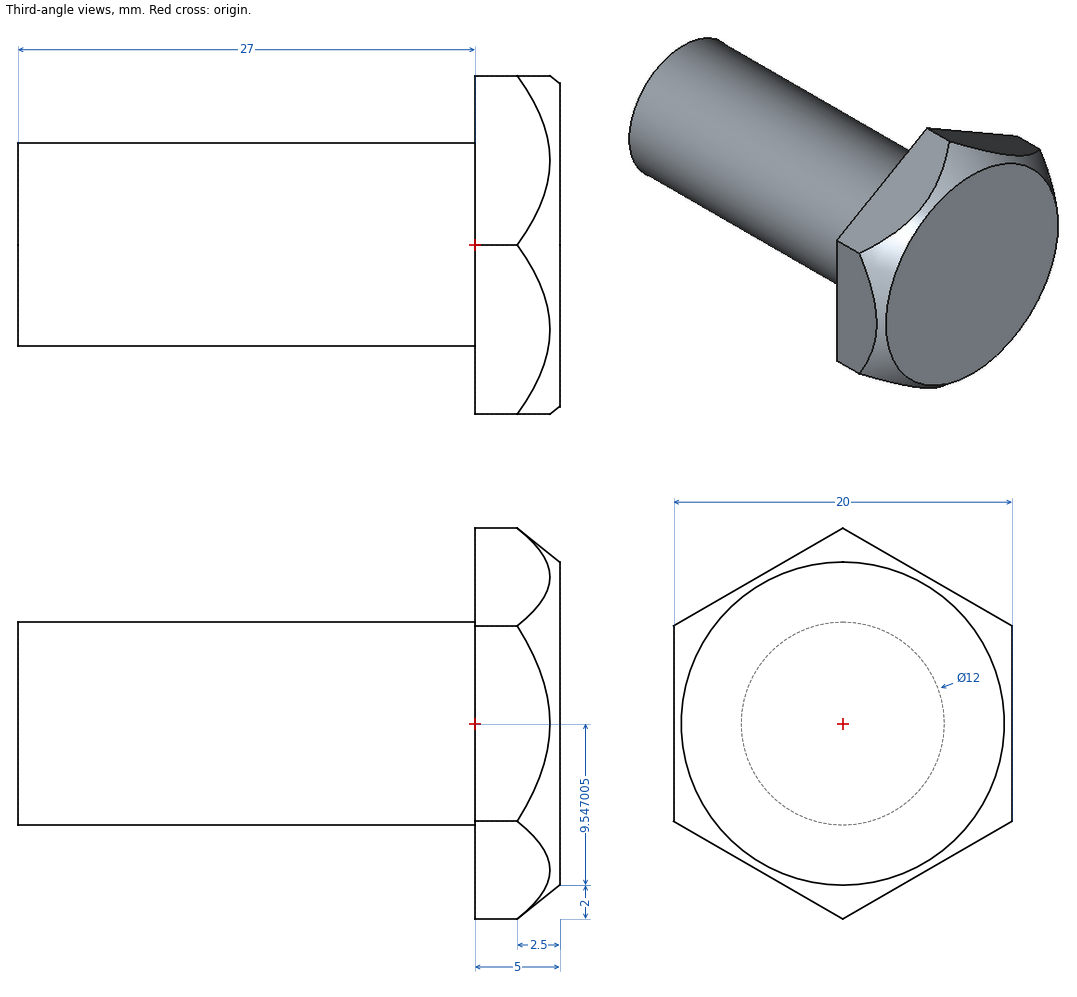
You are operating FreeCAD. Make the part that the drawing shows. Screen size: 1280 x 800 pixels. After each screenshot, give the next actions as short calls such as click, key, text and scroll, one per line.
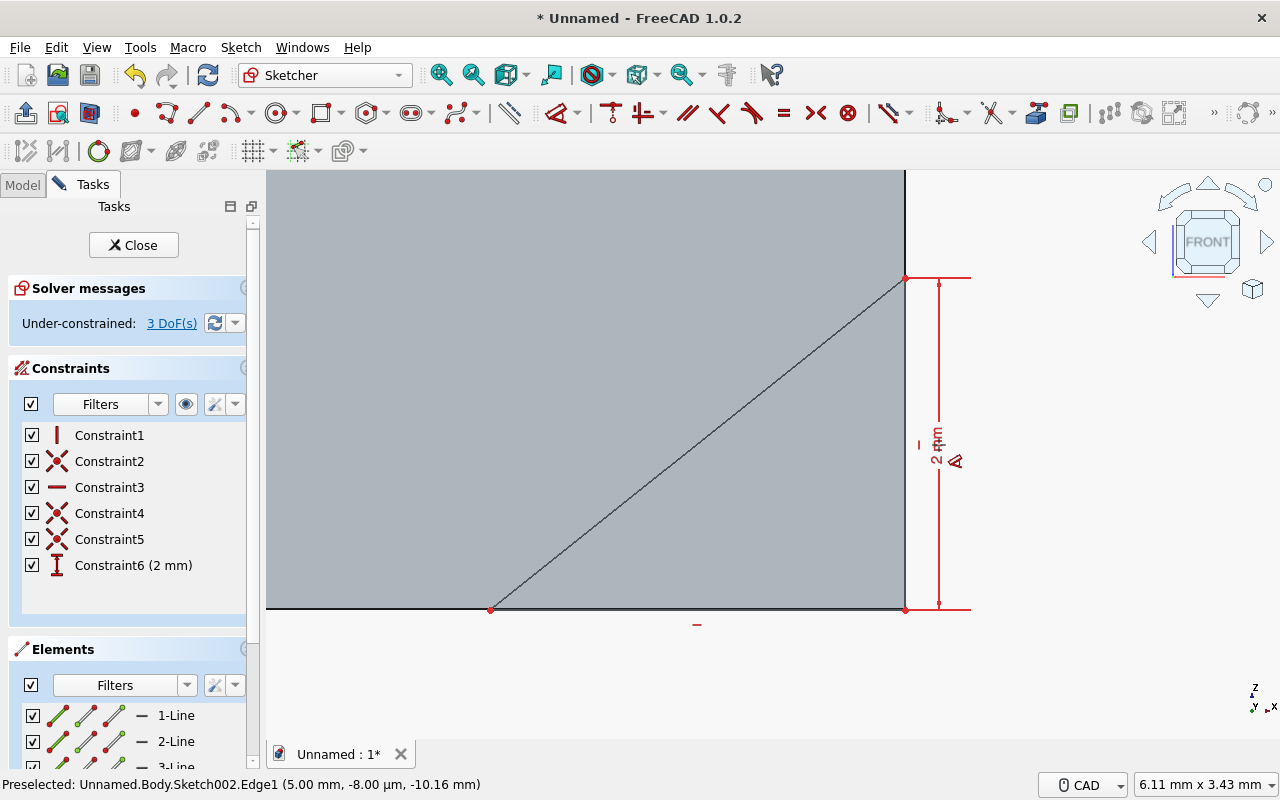
click(905, 278)
click(600, 312)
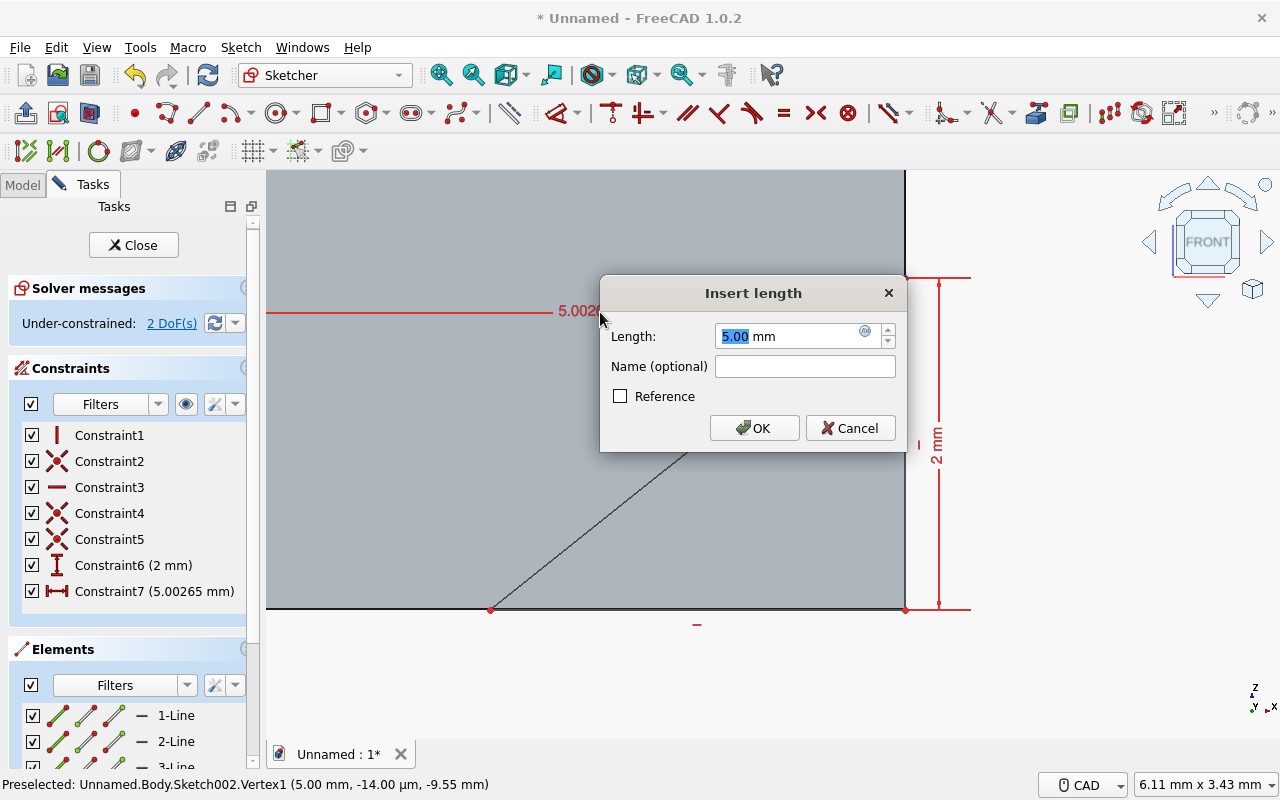
text(5)
key(Return)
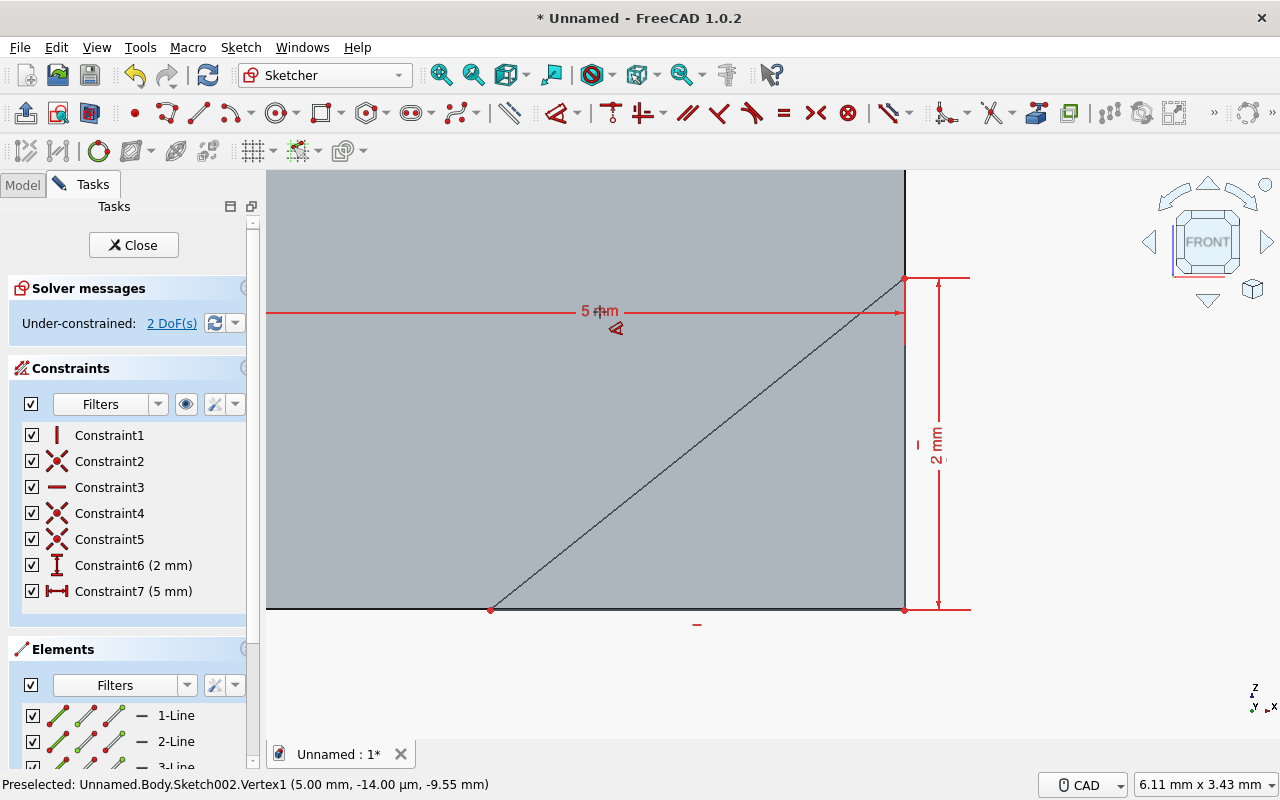
click(780, 610)
click(697, 644)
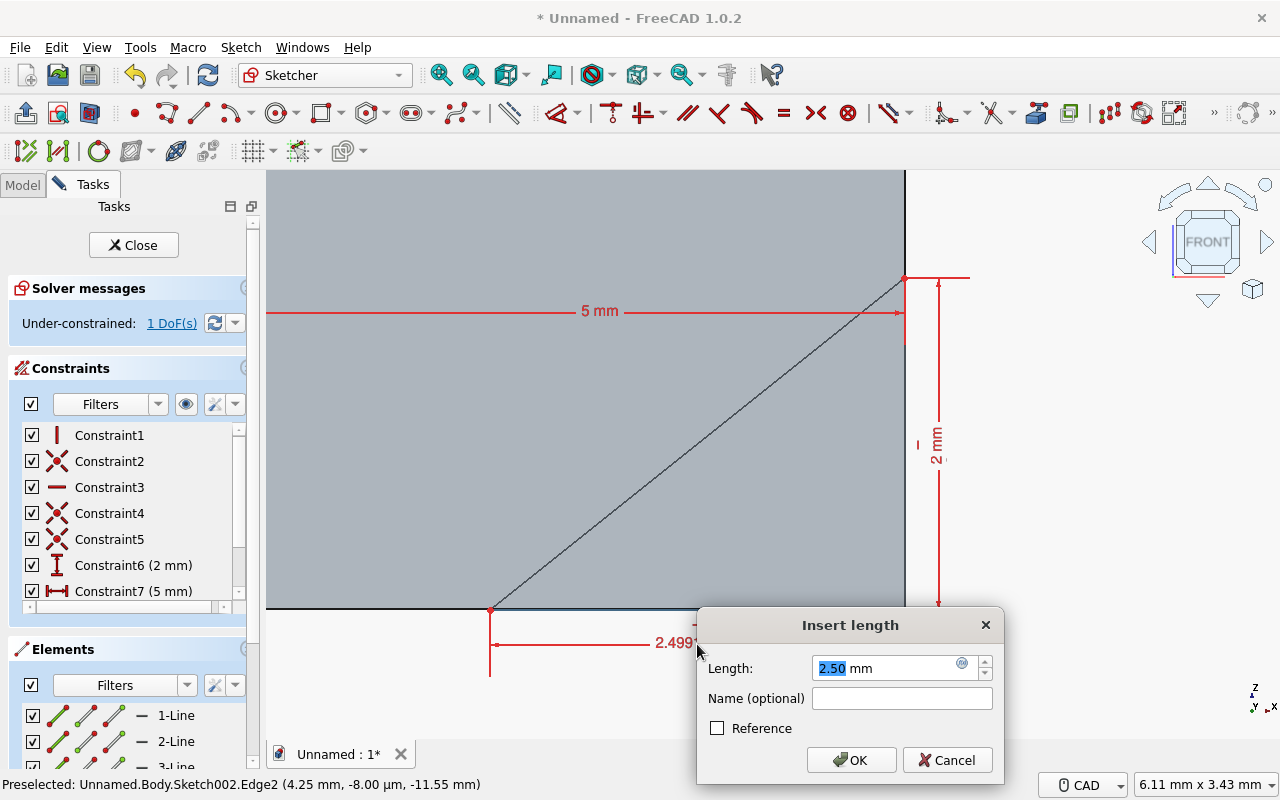
text(2.5)
key(Return)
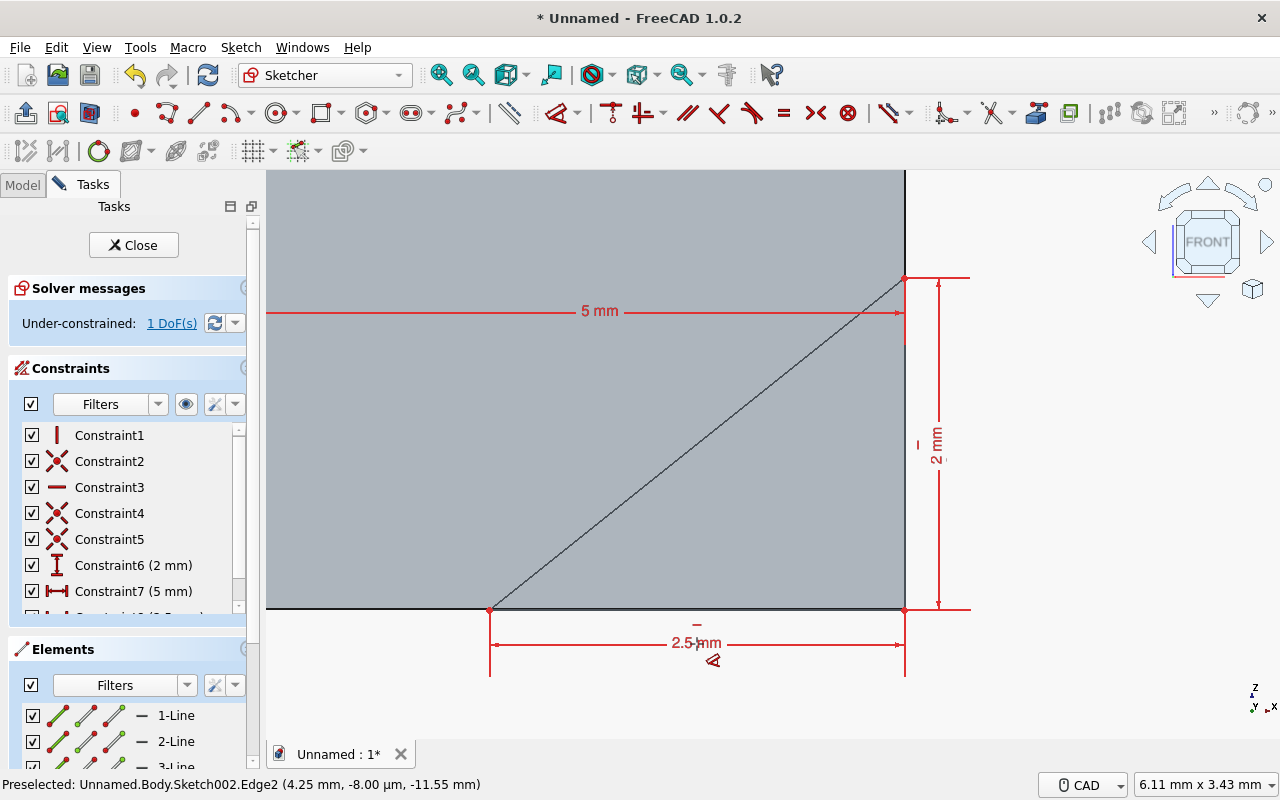
click(905, 278)
click(939, 238)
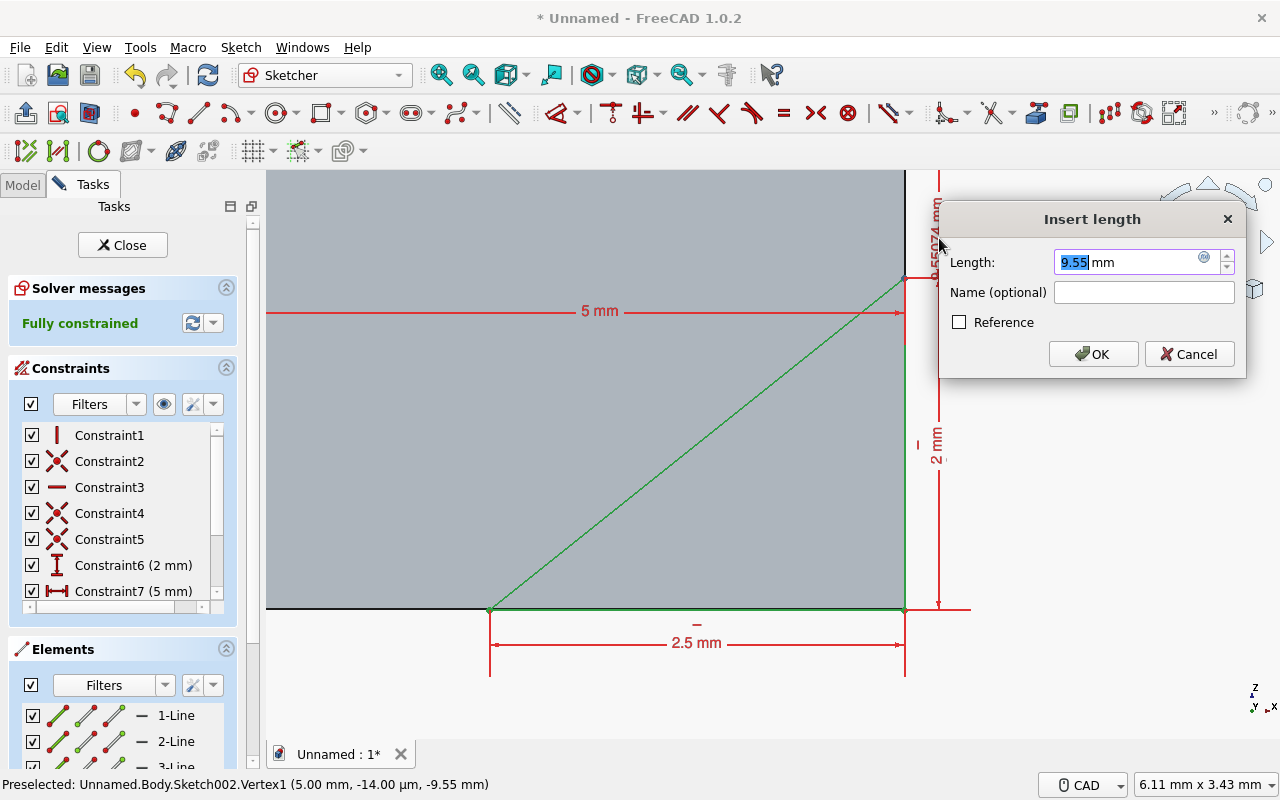
text(9.547005)
key(Return)
key(Escape)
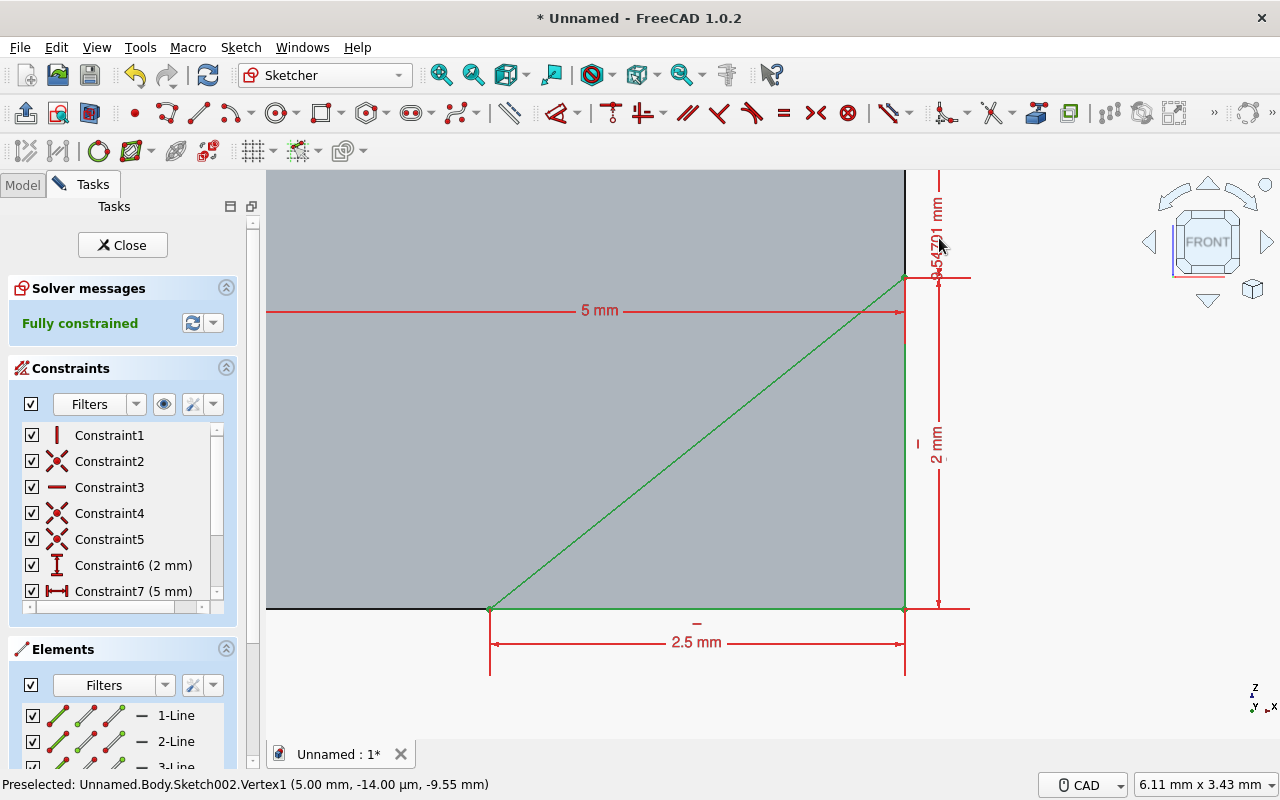
click(123, 245)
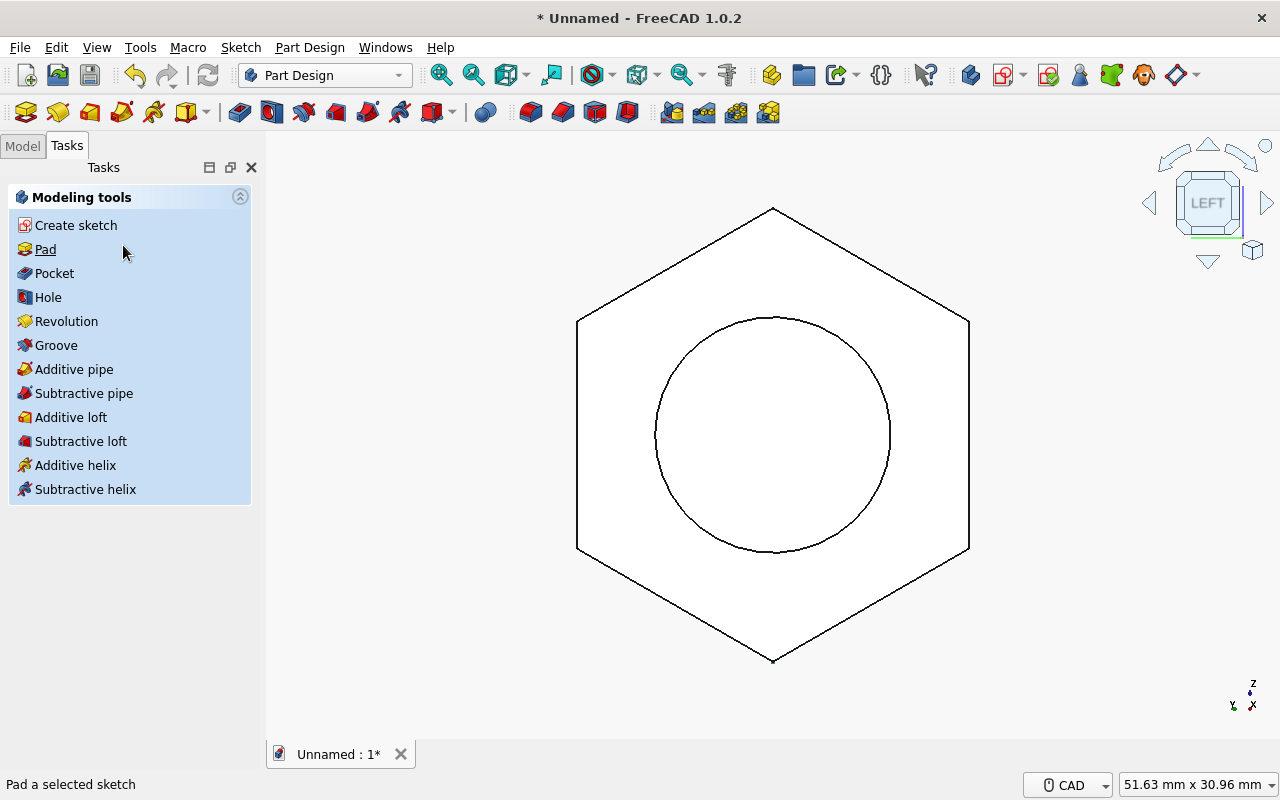
click(304, 112)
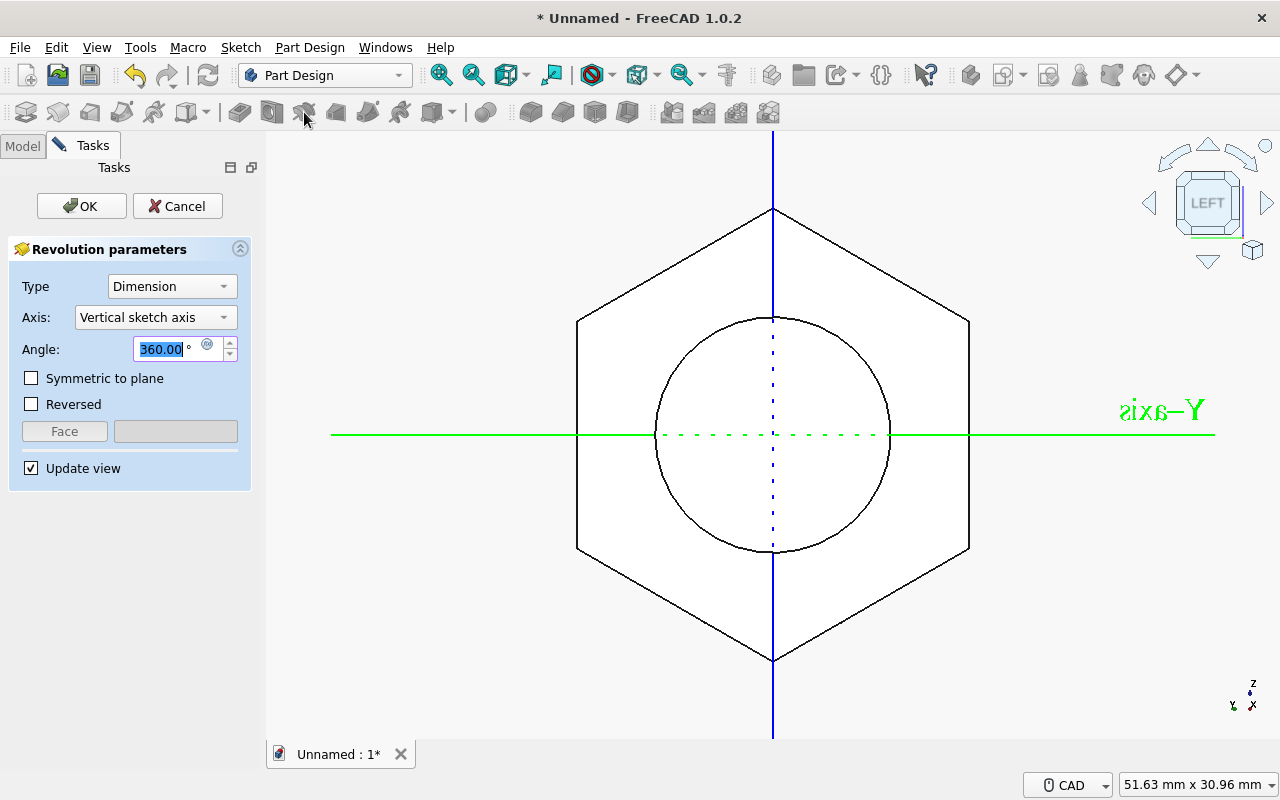
click(156, 318)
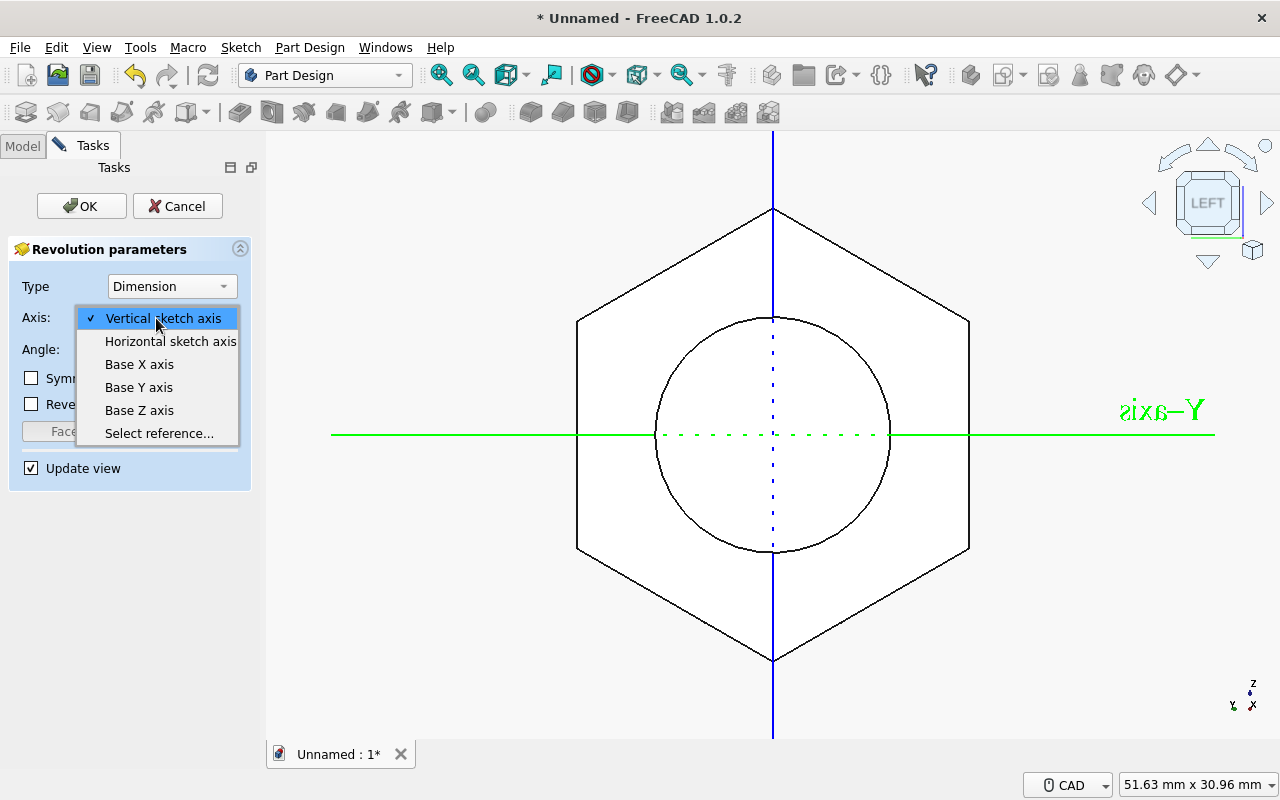
click(156, 342)